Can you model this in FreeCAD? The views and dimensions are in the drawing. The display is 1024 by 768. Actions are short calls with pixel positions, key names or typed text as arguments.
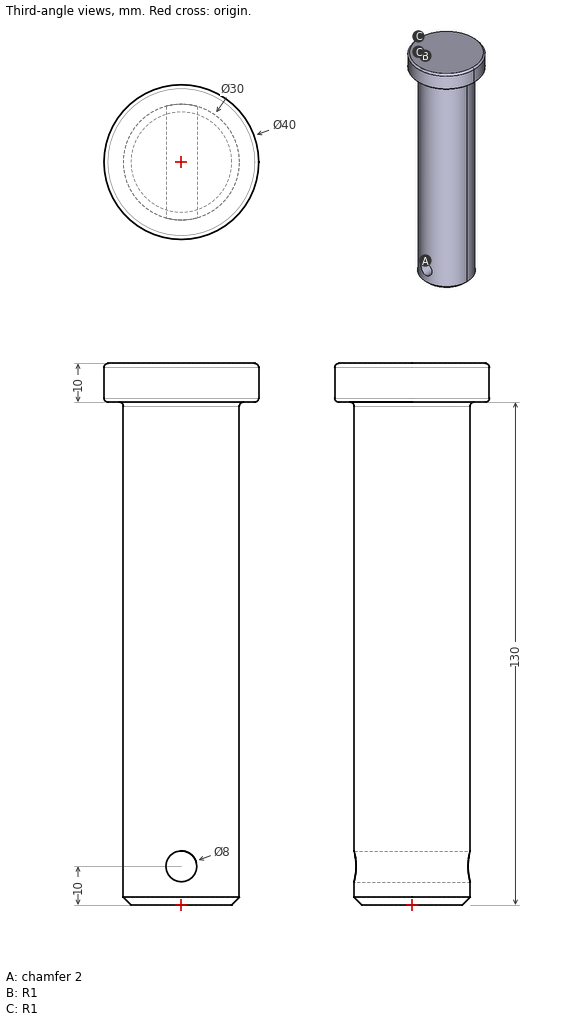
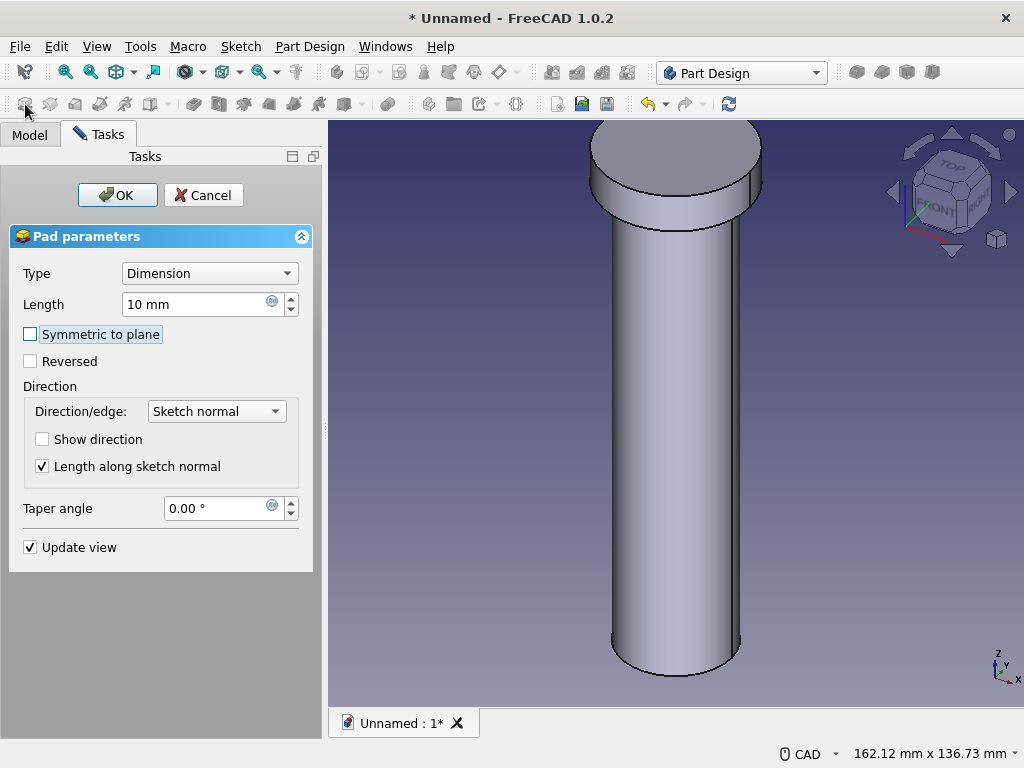
click(118, 195)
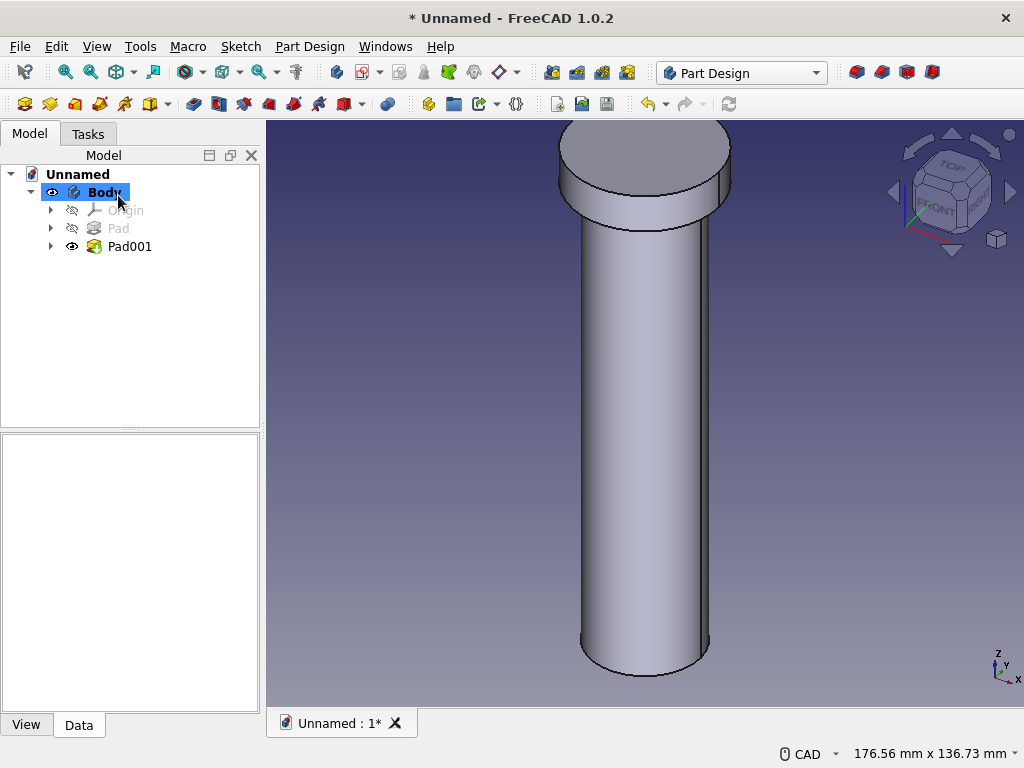
click(66, 72)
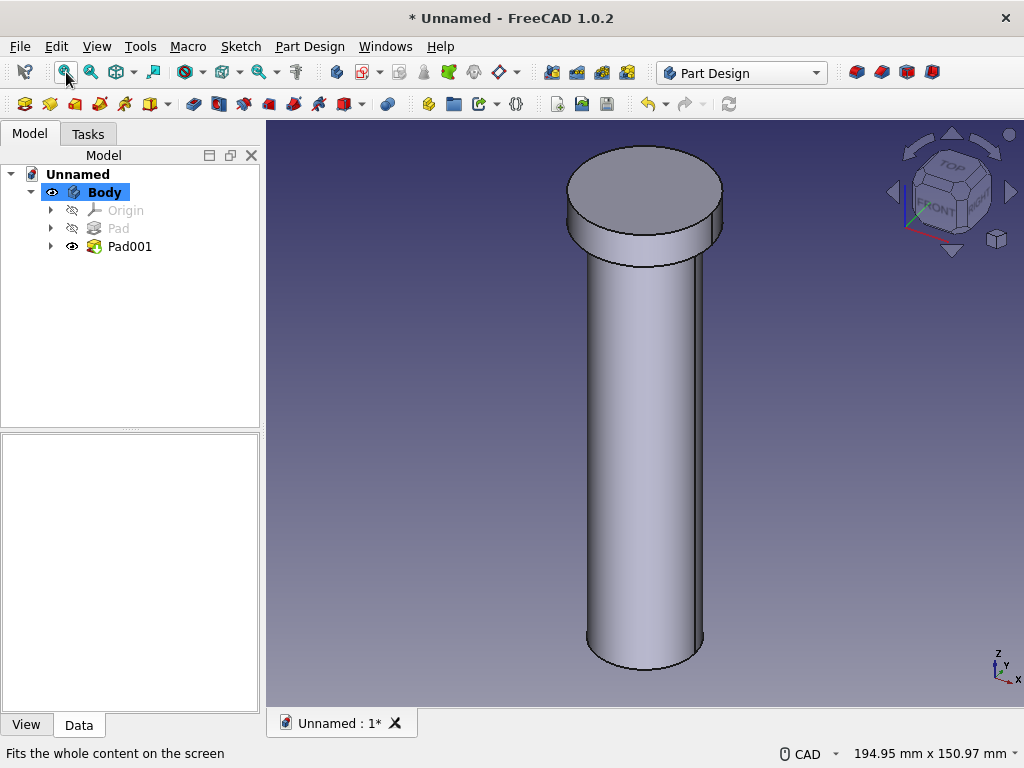
click(362, 72)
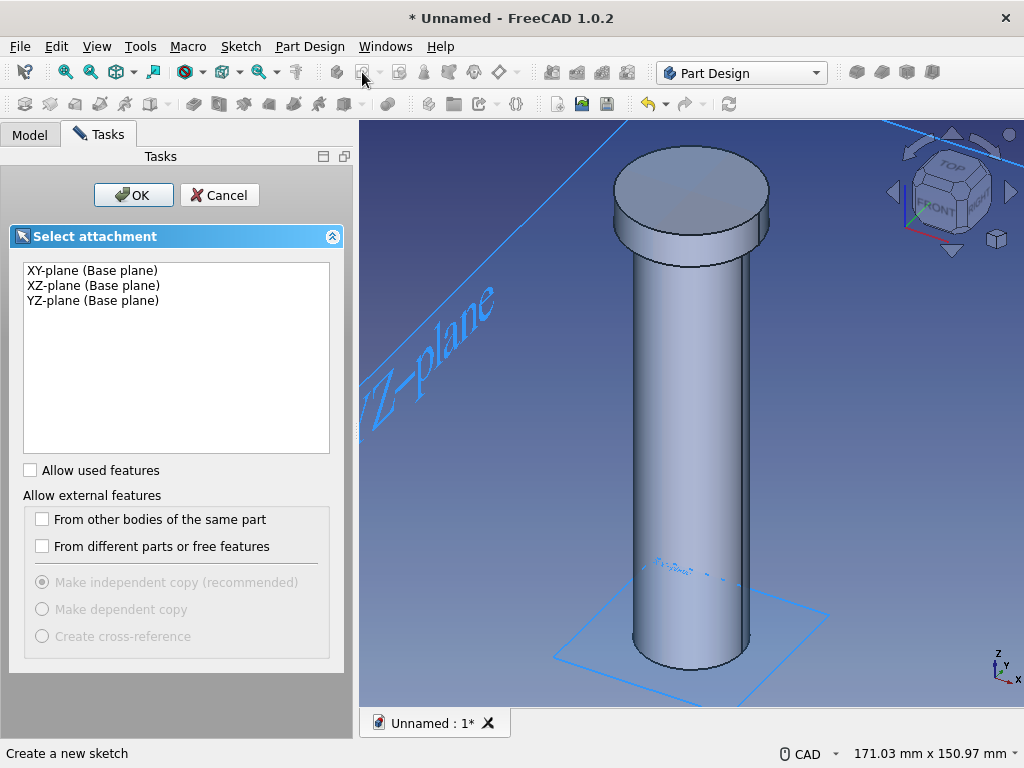
click(84, 286)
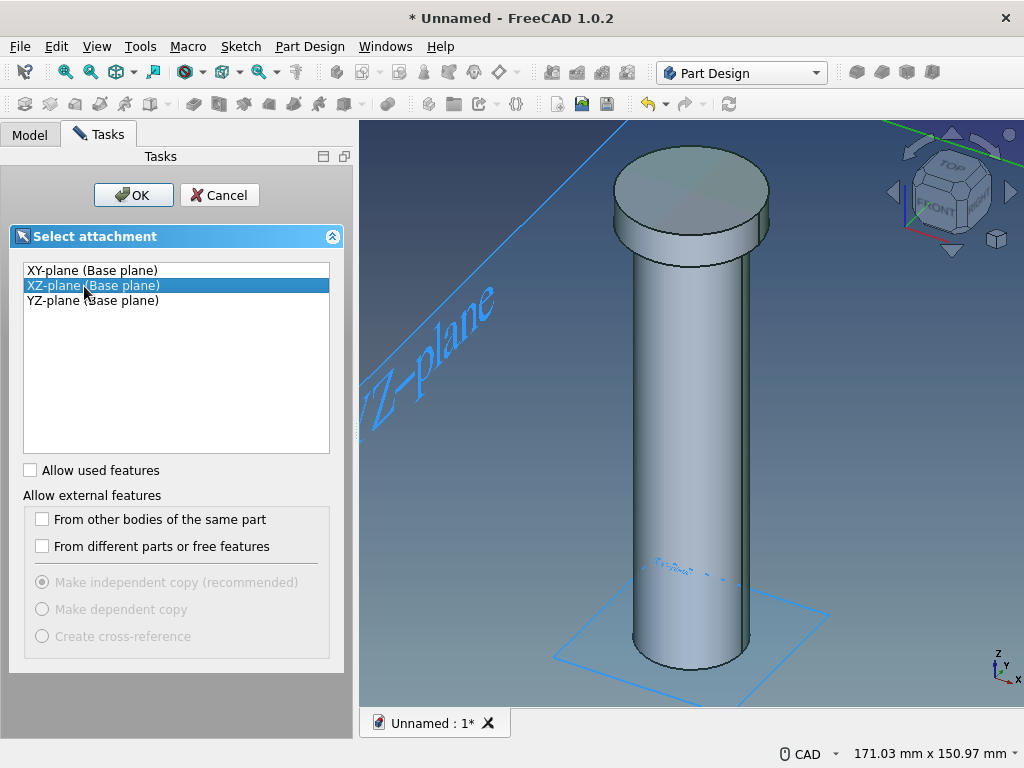
click(134, 195)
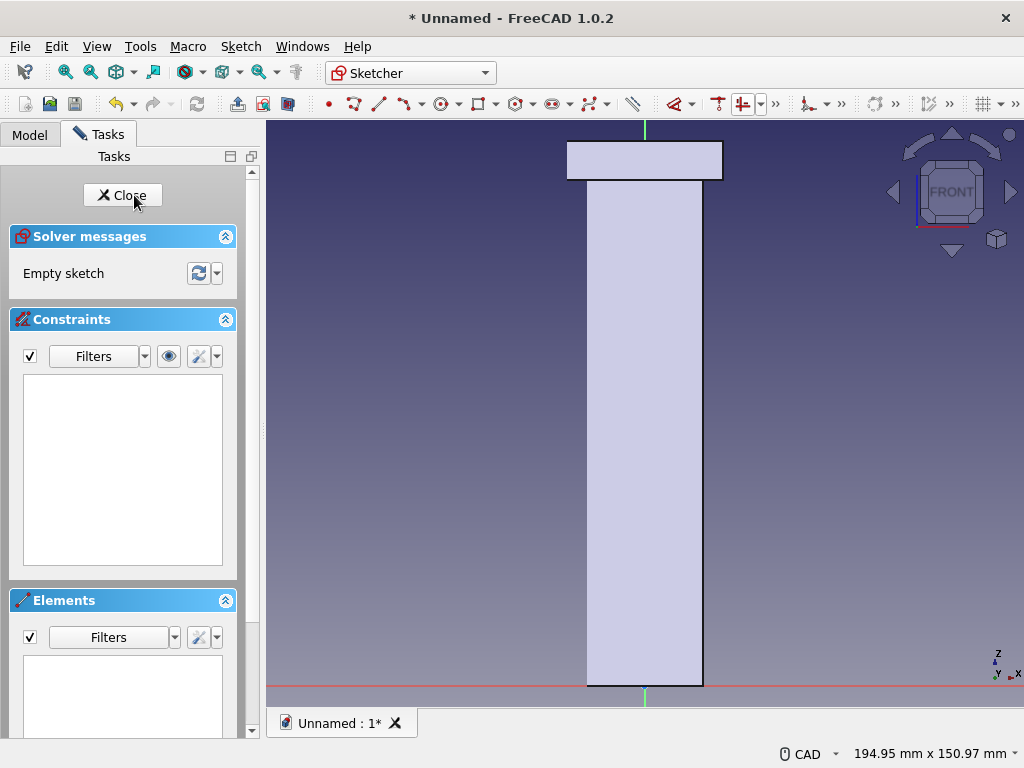
click(288, 104)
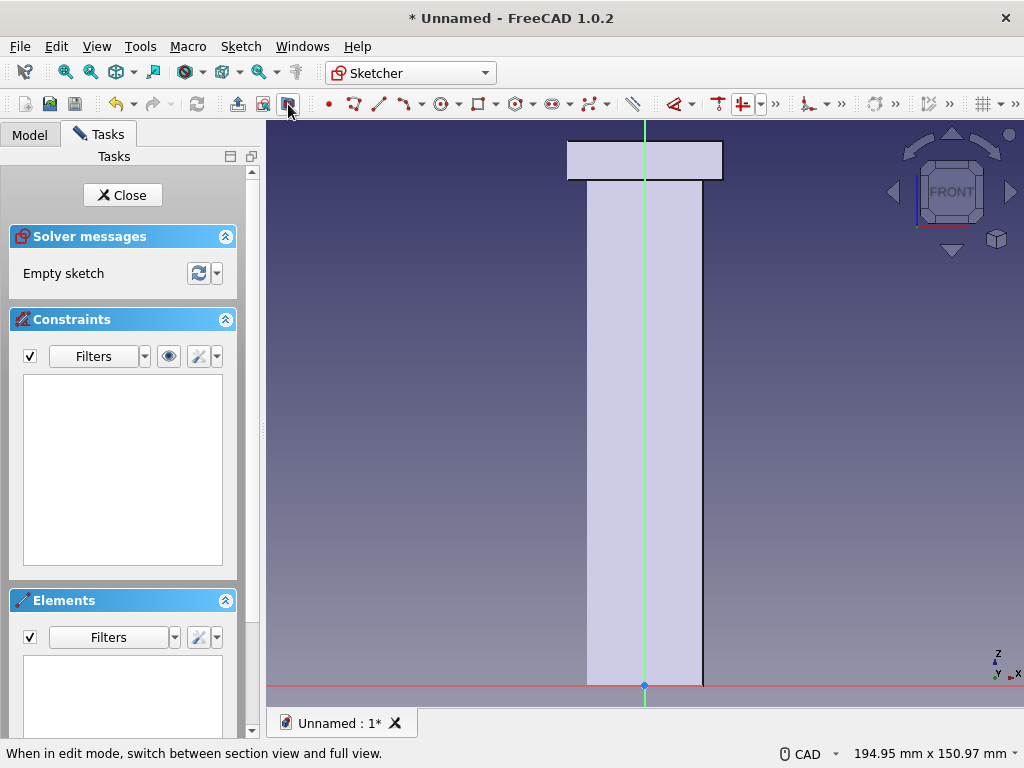
scroll(576, 414, down, 5)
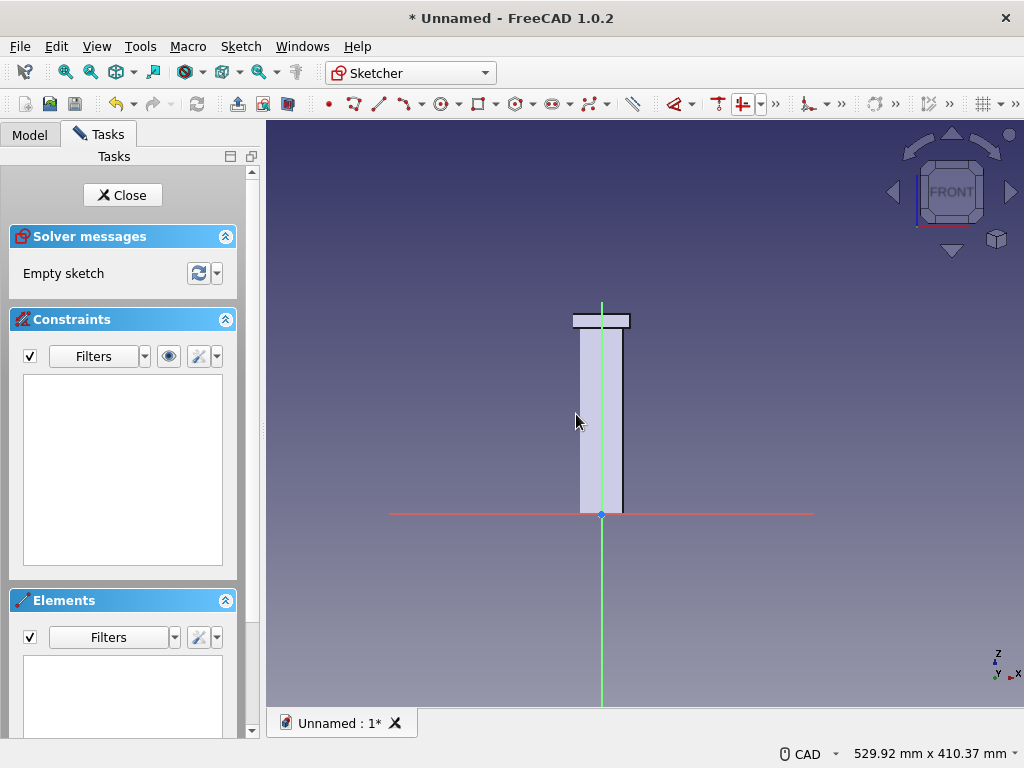
scroll(603, 509, up, 15)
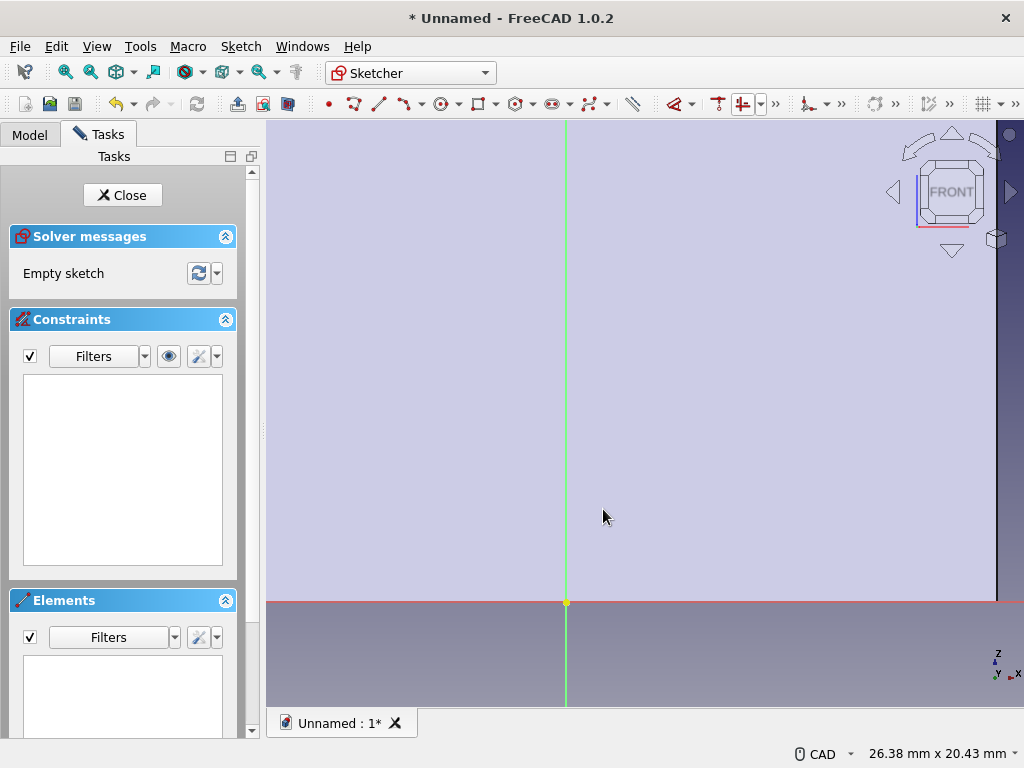
click(440, 104)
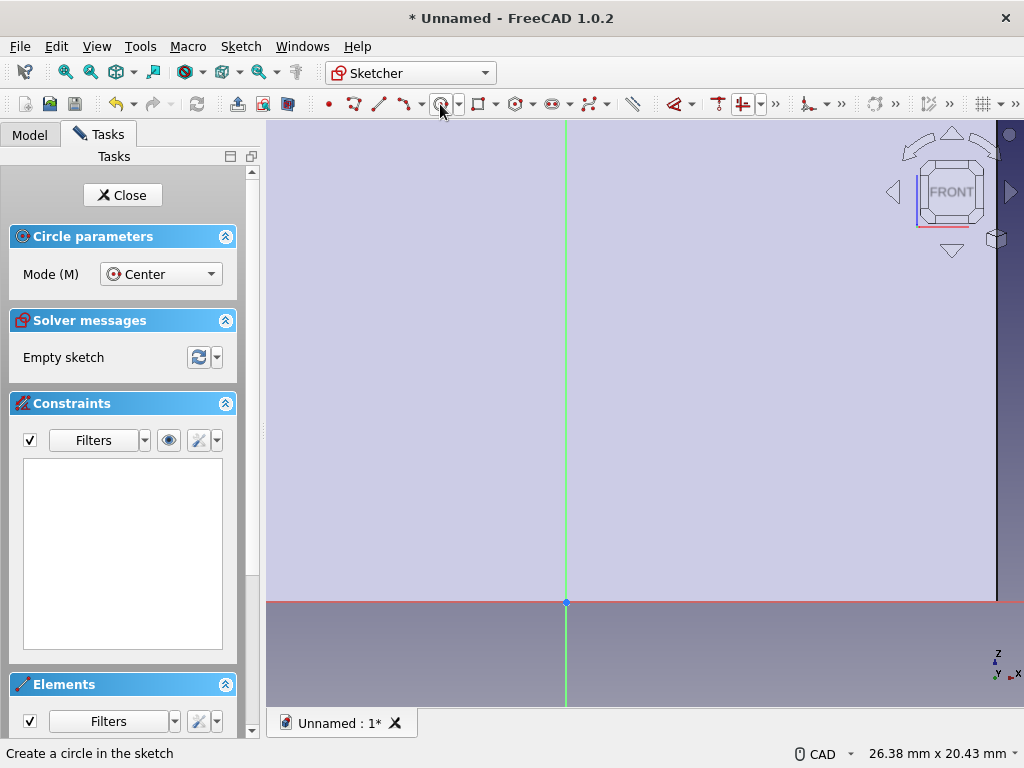
click(566, 315)
click(647, 233)
key(Escape)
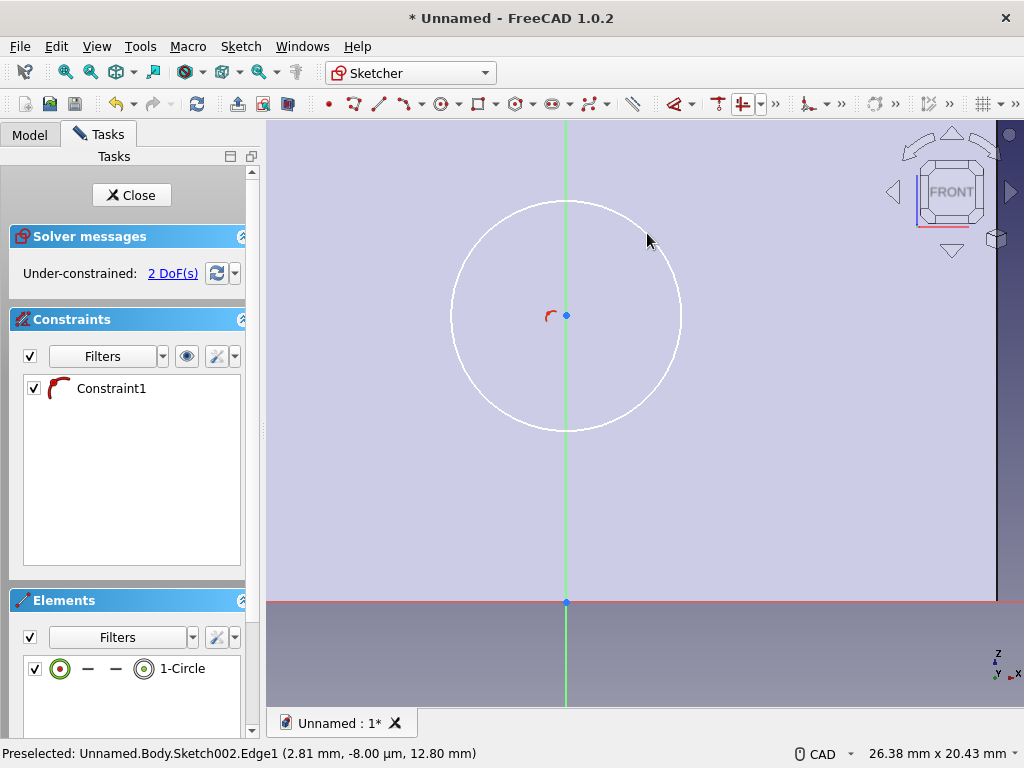
click(674, 104)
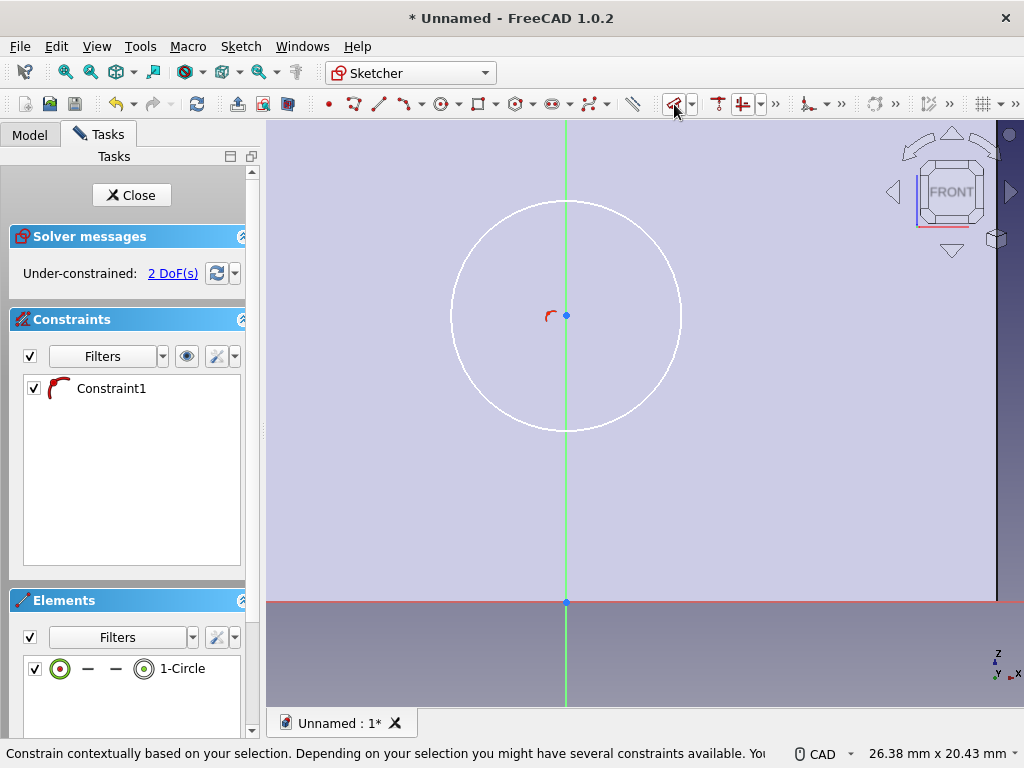
click(647, 234)
click(669, 211)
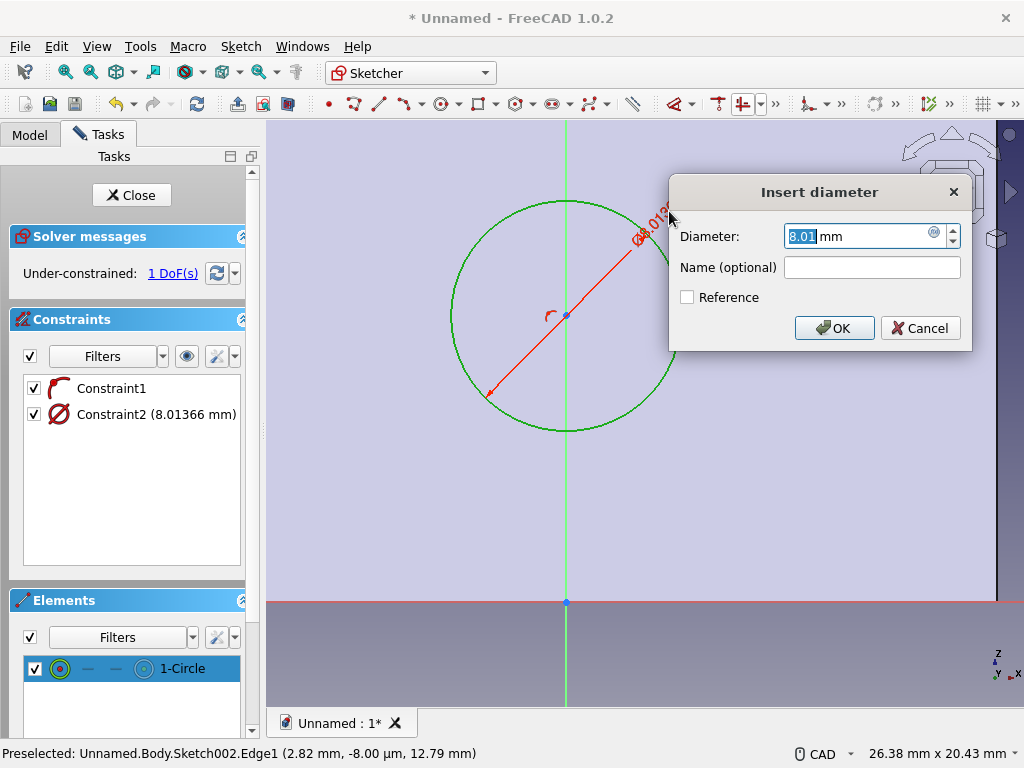
text(8)
key(Return)